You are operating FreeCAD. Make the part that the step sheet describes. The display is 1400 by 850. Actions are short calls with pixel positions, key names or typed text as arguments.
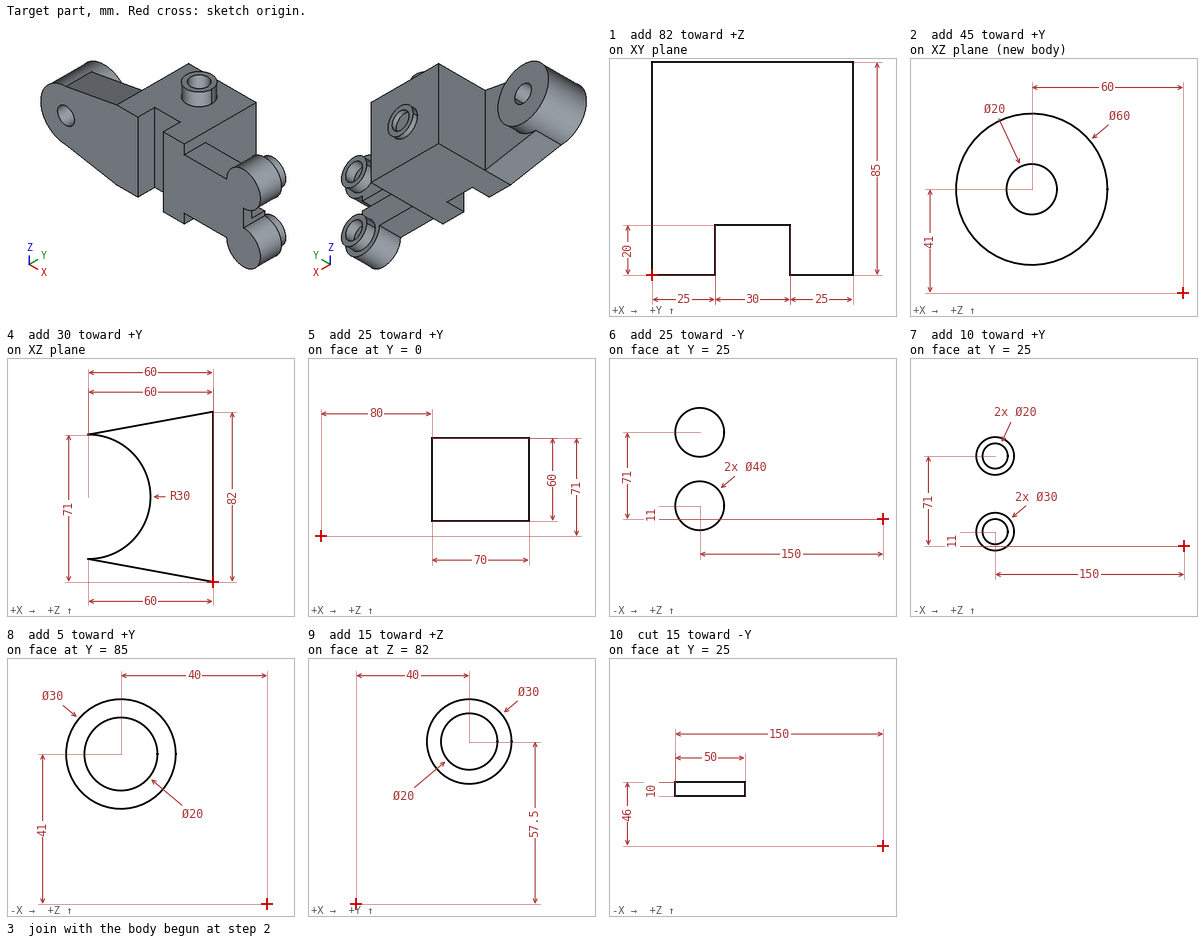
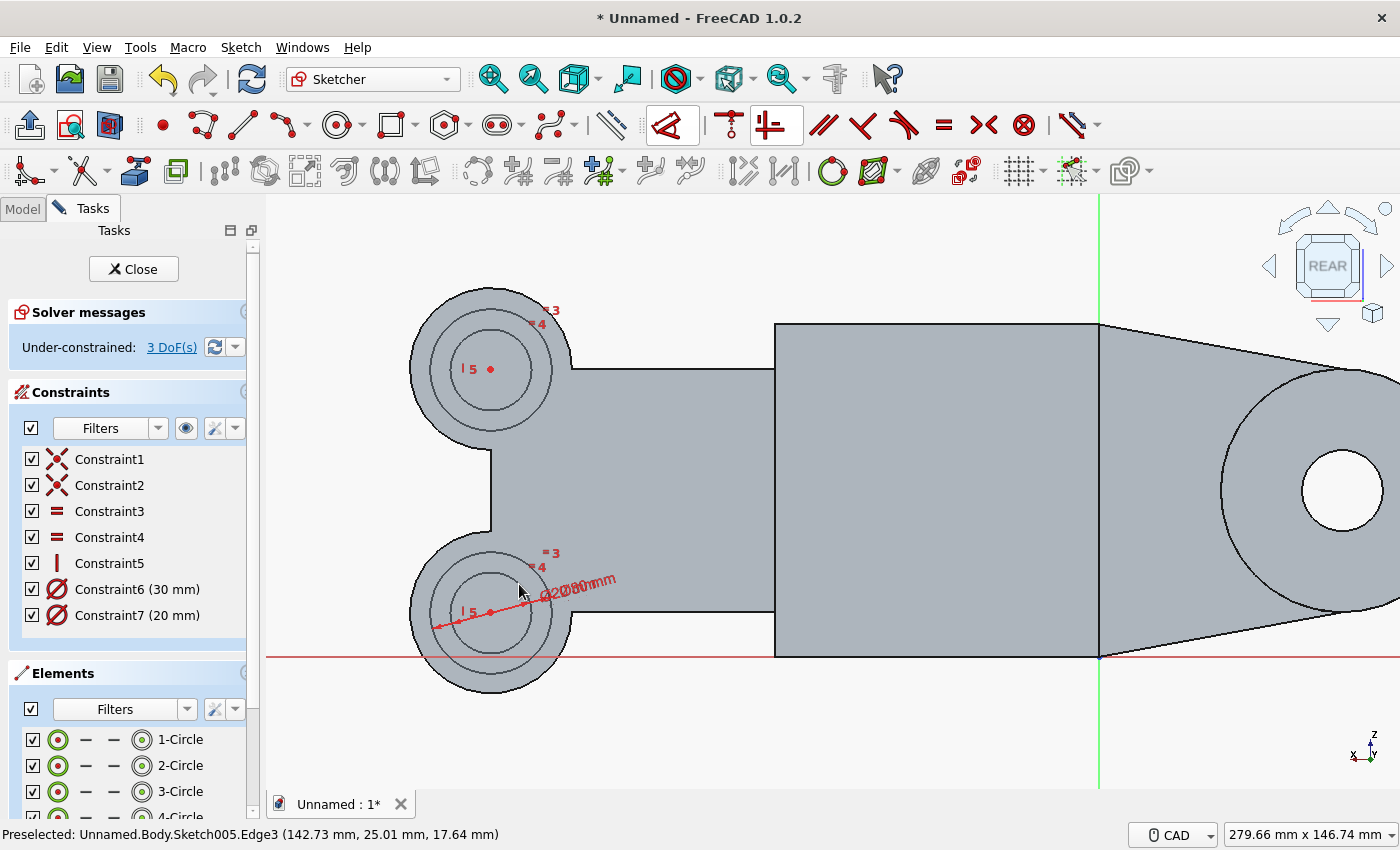
click(491, 613)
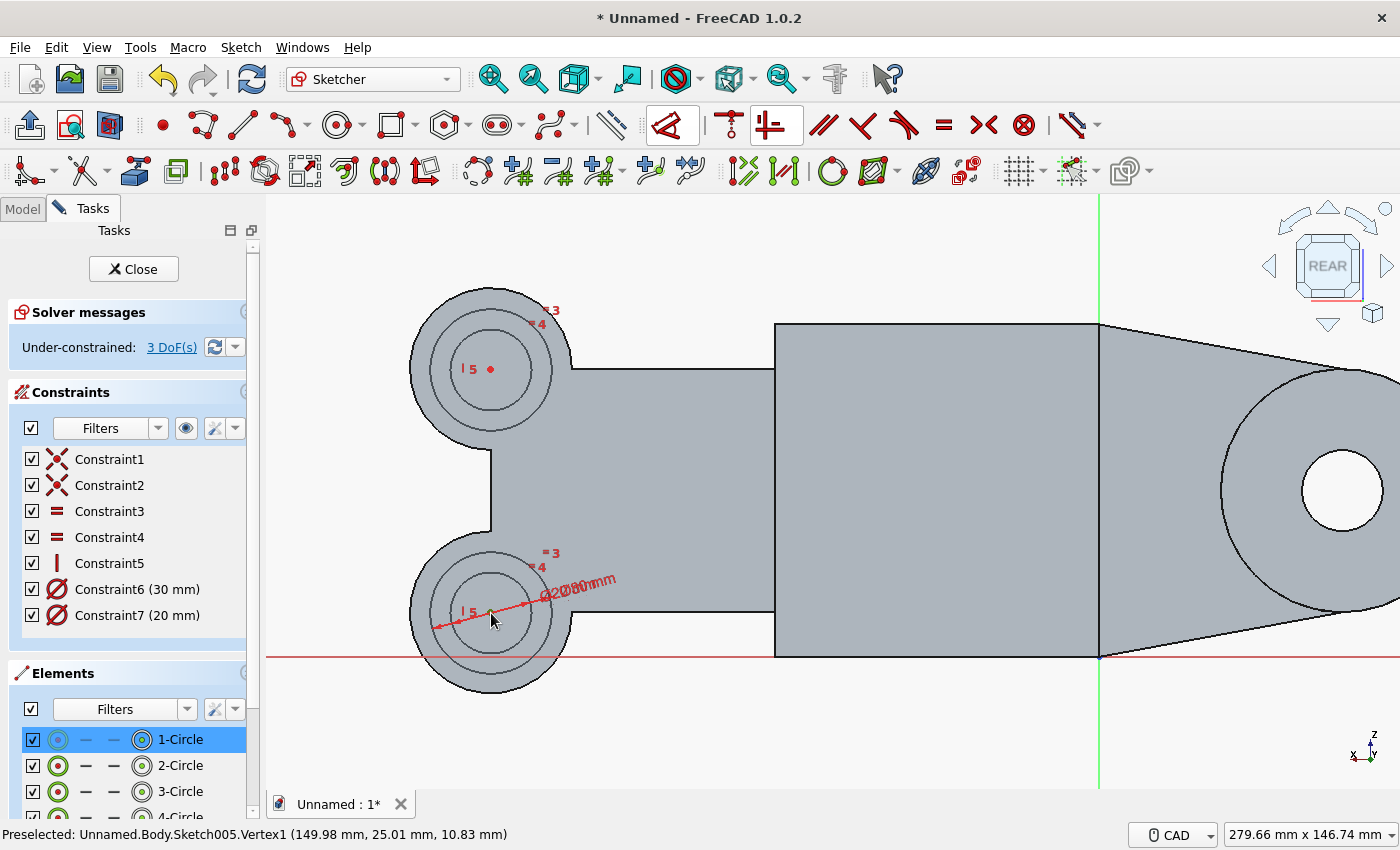
click(694, 126)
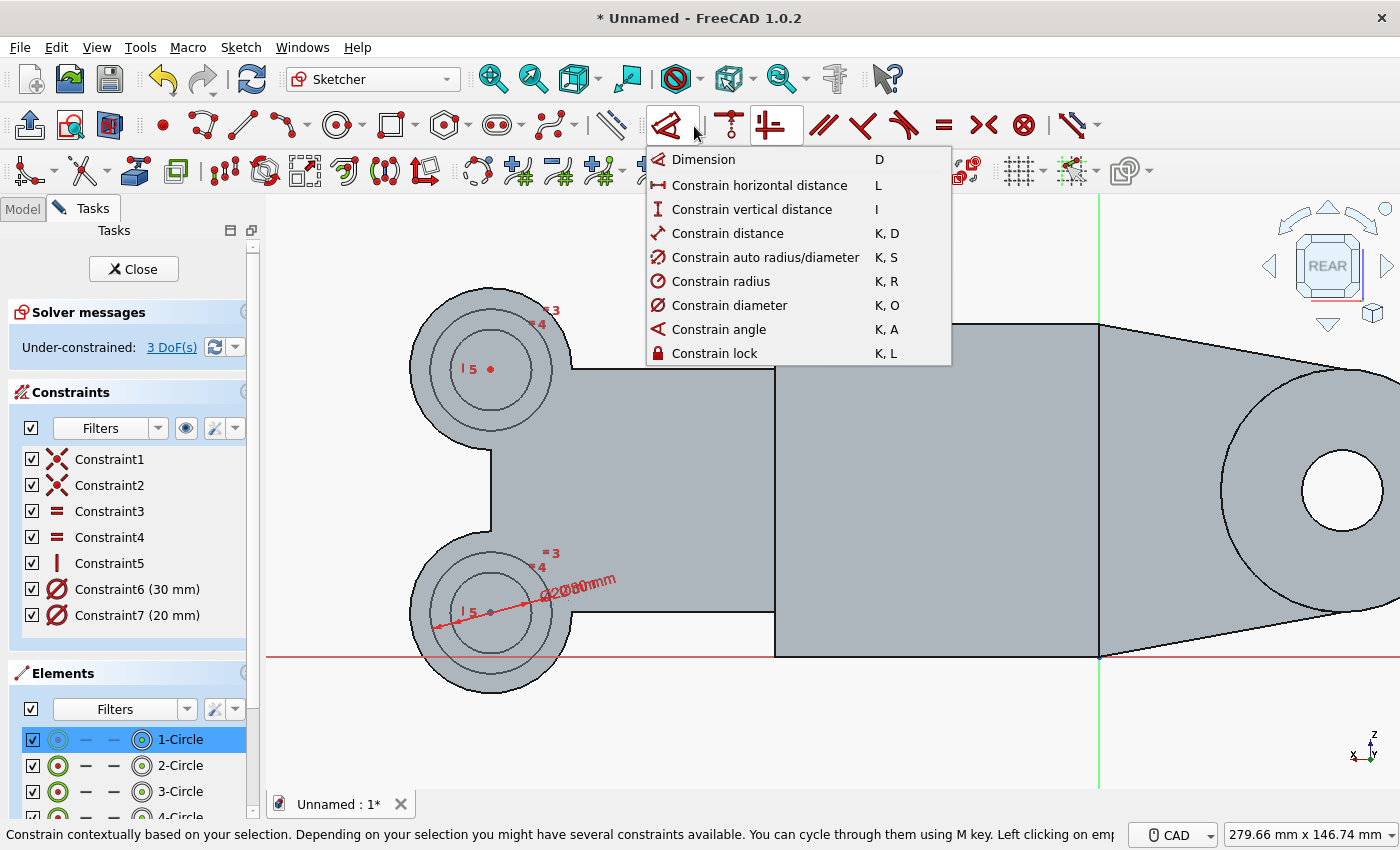
click(799, 209)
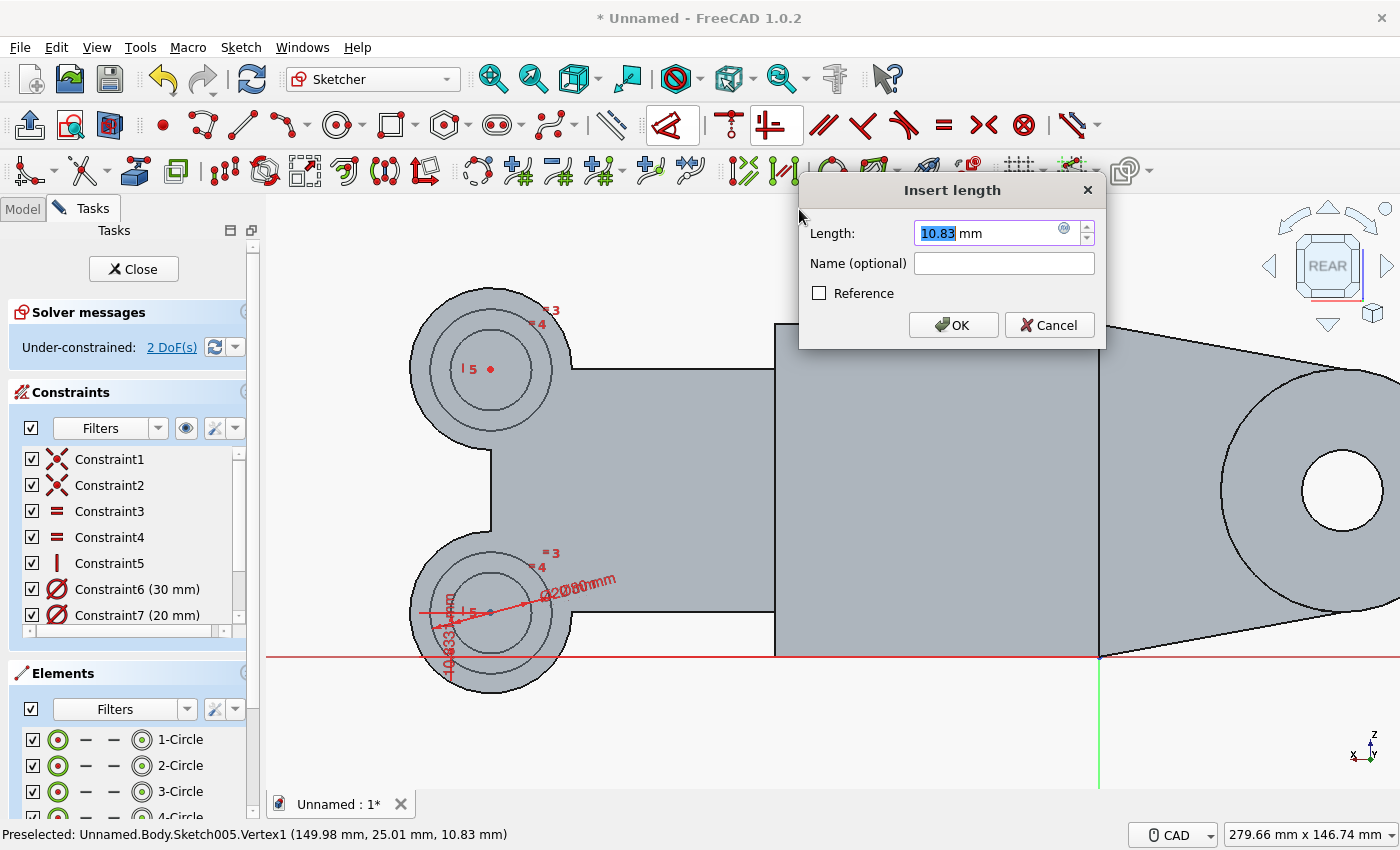
text(11)
key(Return)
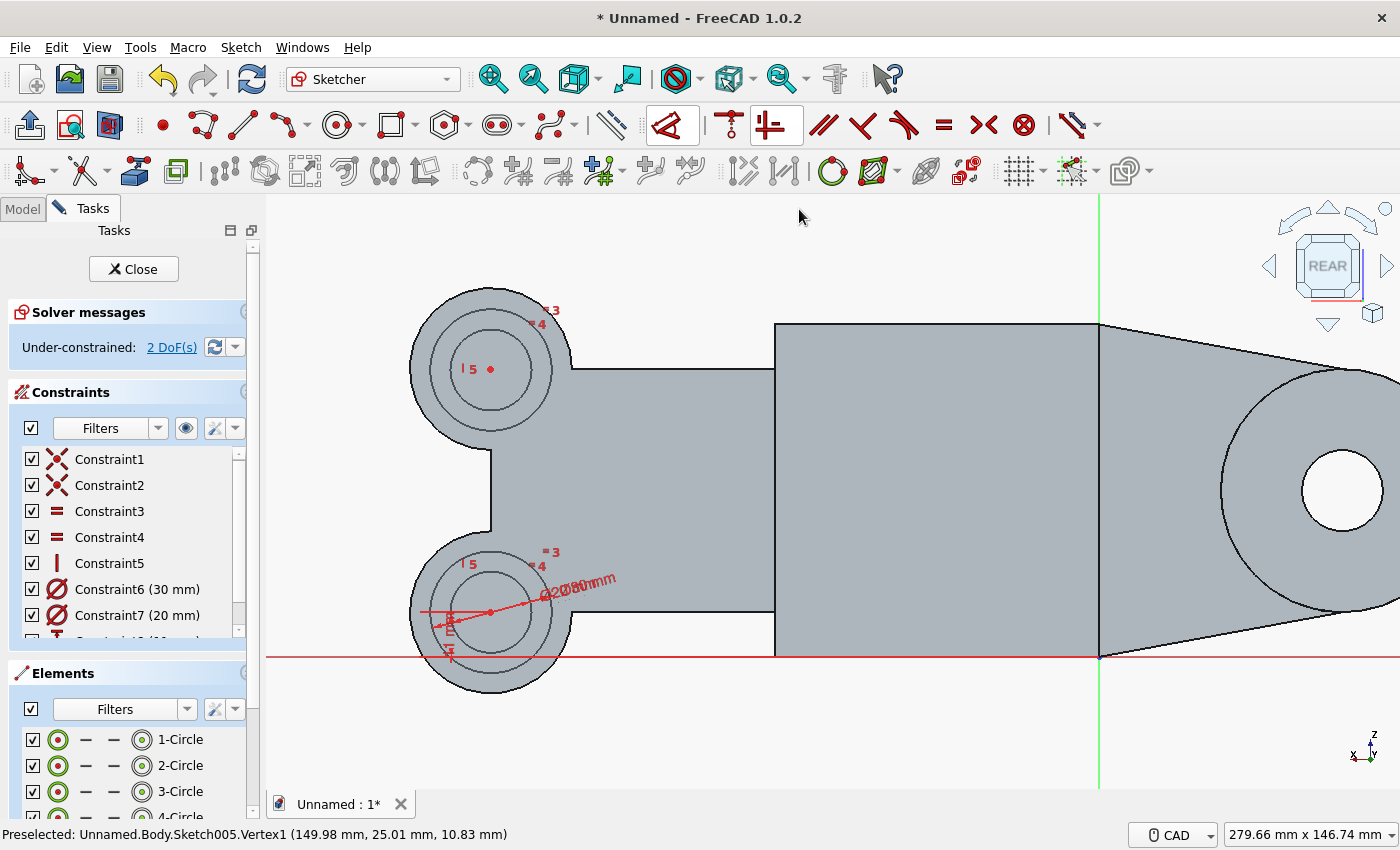
click(491, 370)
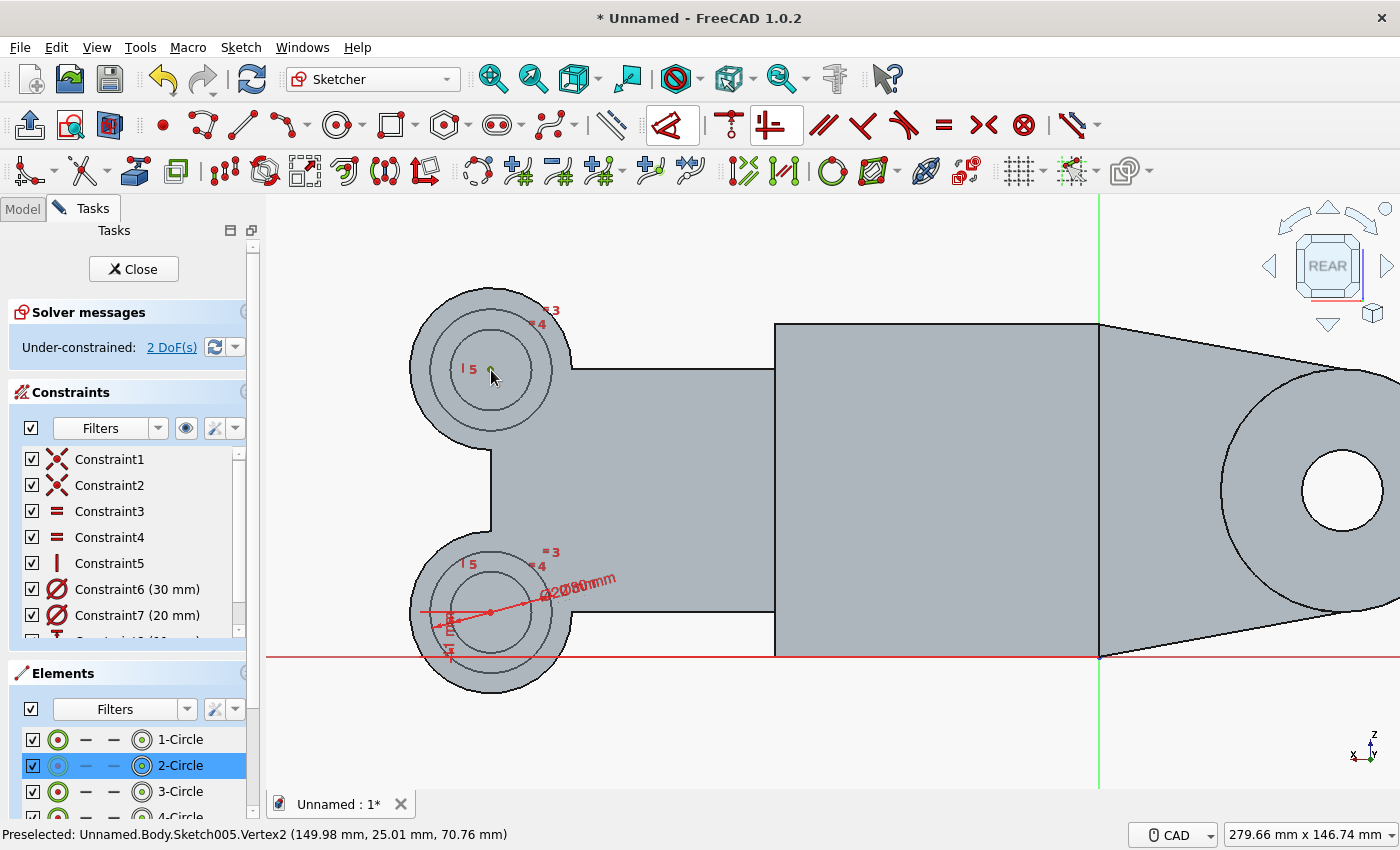
key(i)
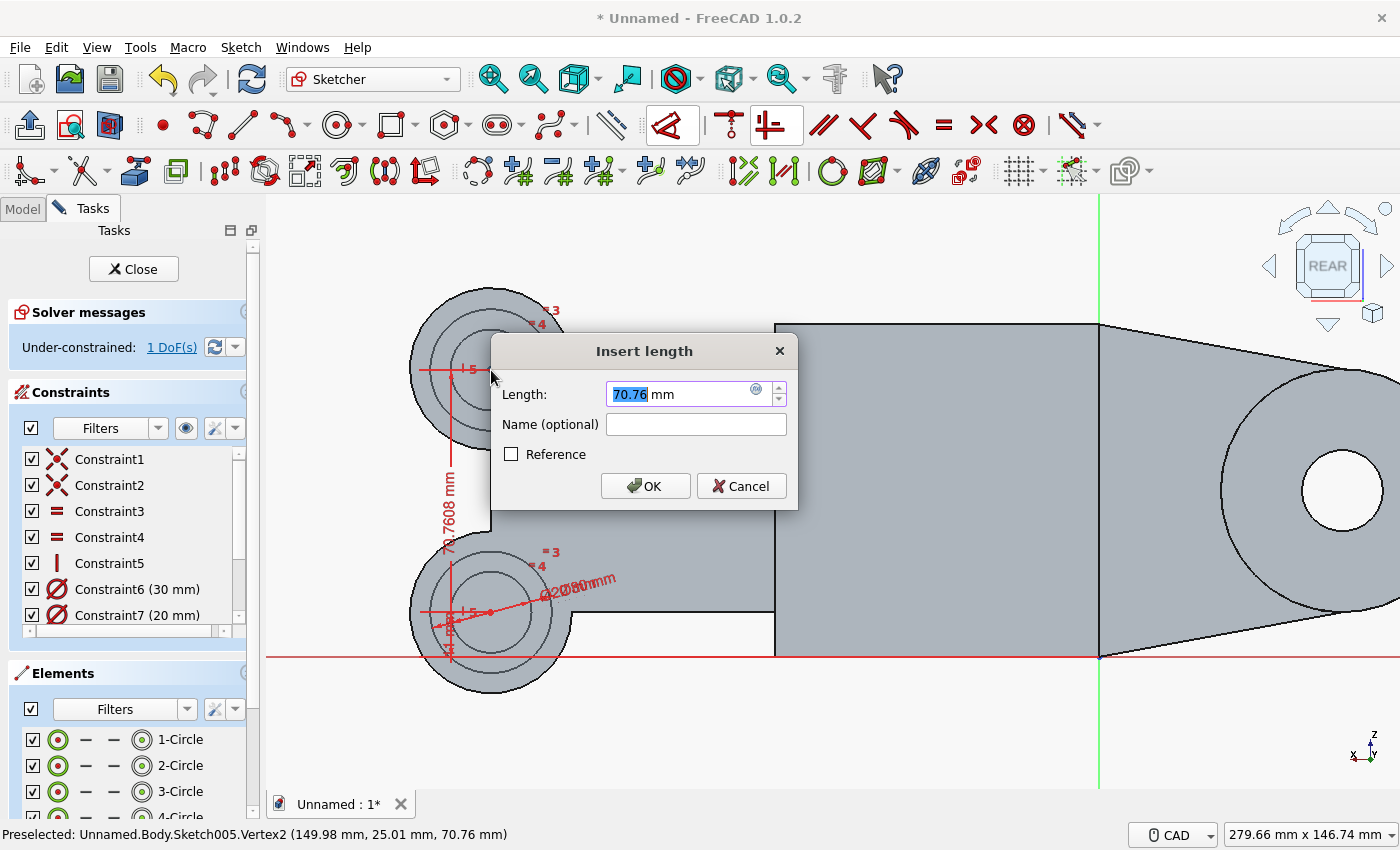
text(71)
key(Return)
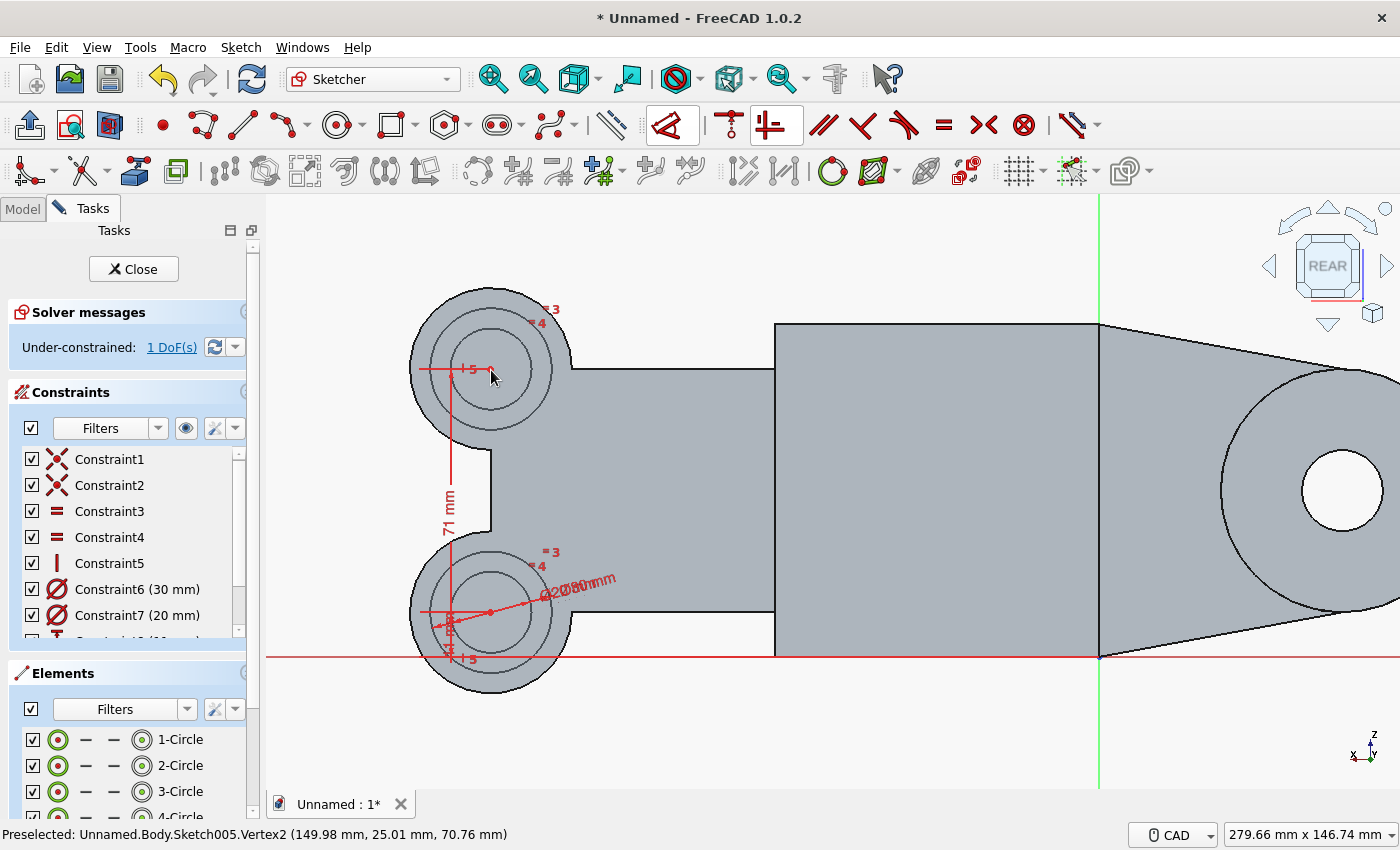
click(491, 612)